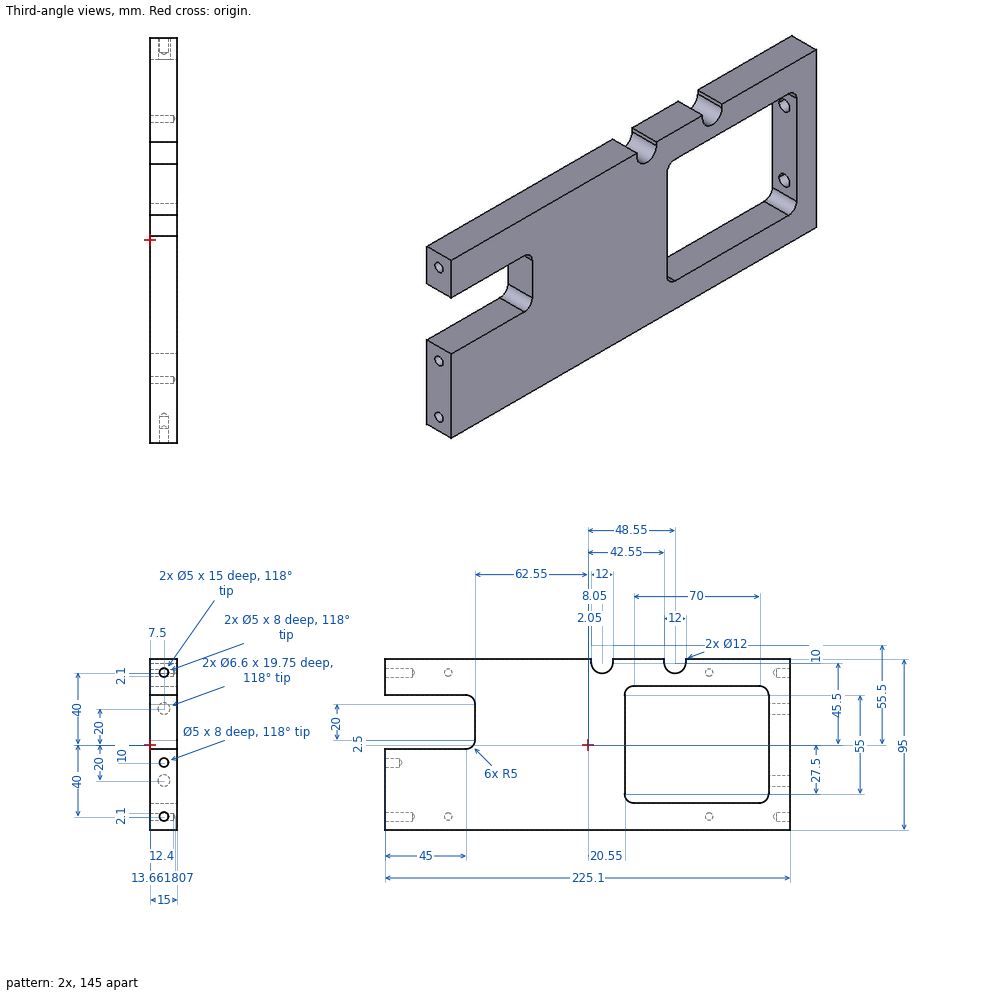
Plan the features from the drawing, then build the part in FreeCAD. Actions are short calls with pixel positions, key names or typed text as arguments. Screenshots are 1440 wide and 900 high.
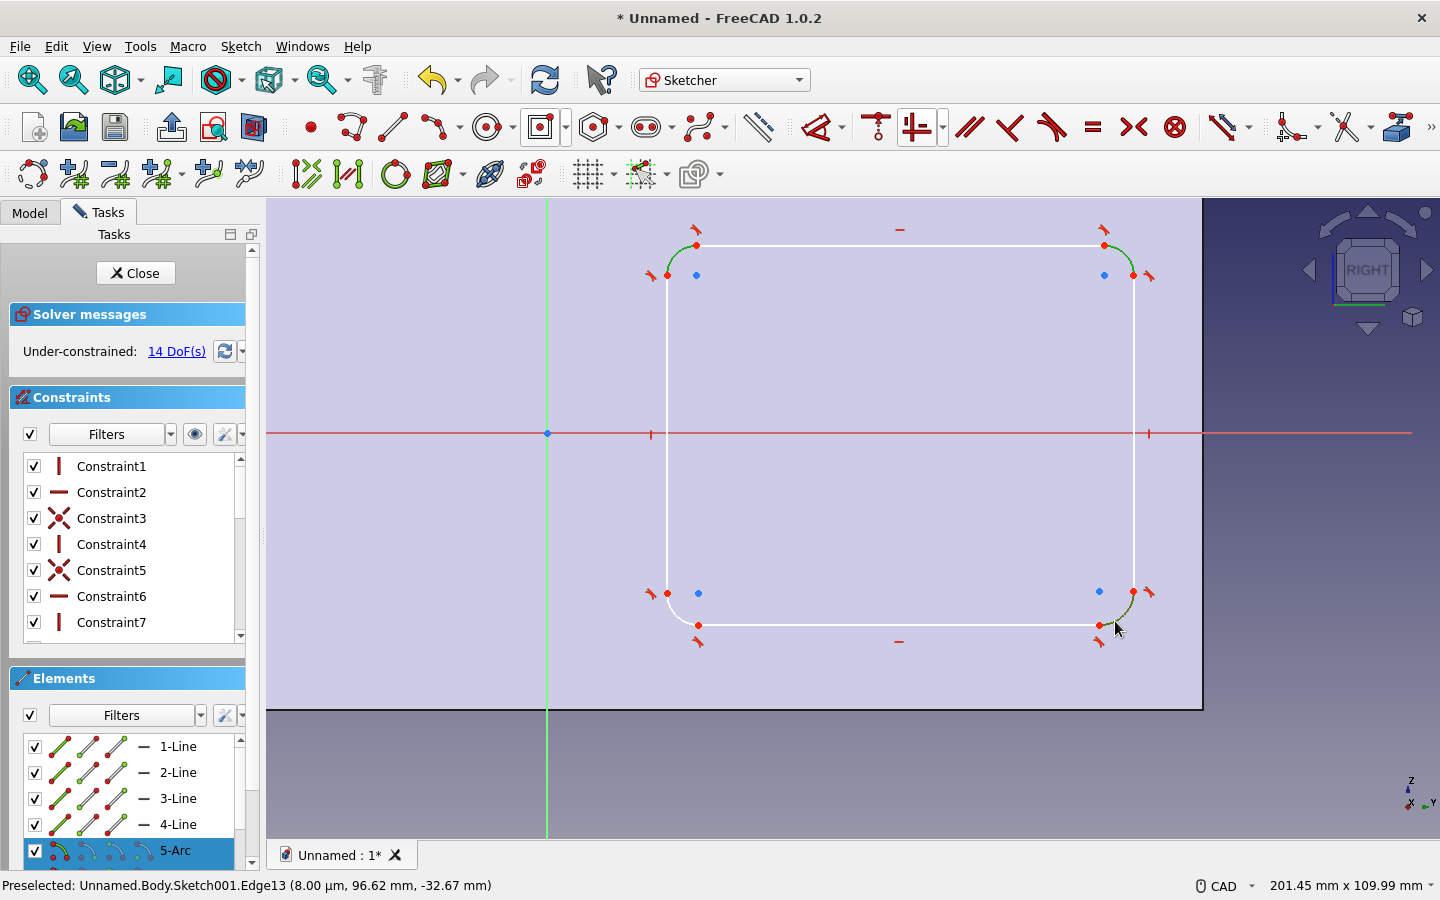
click(671, 608)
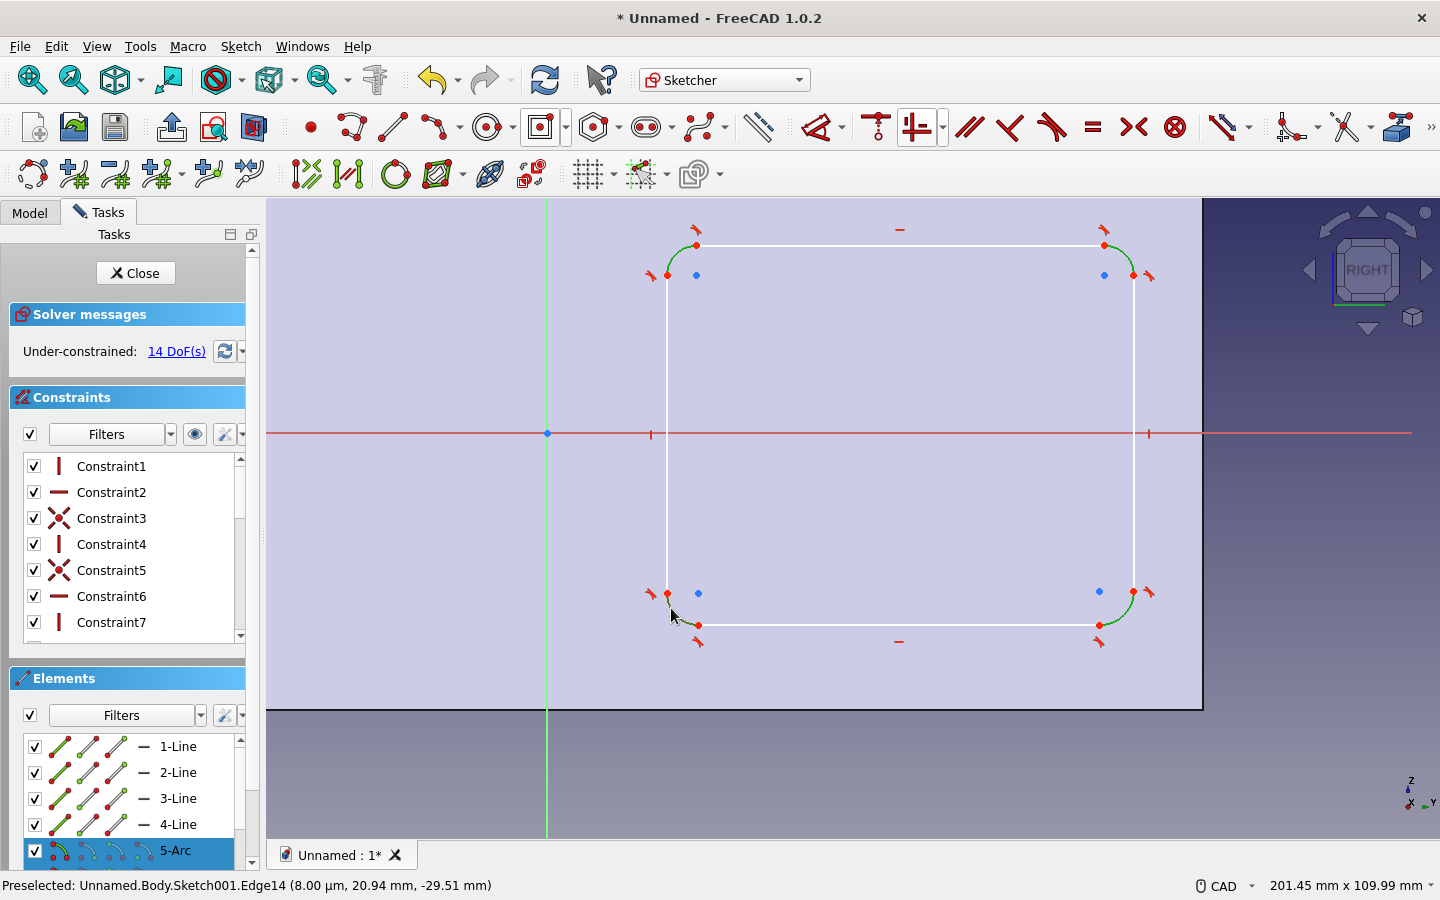
click(1093, 128)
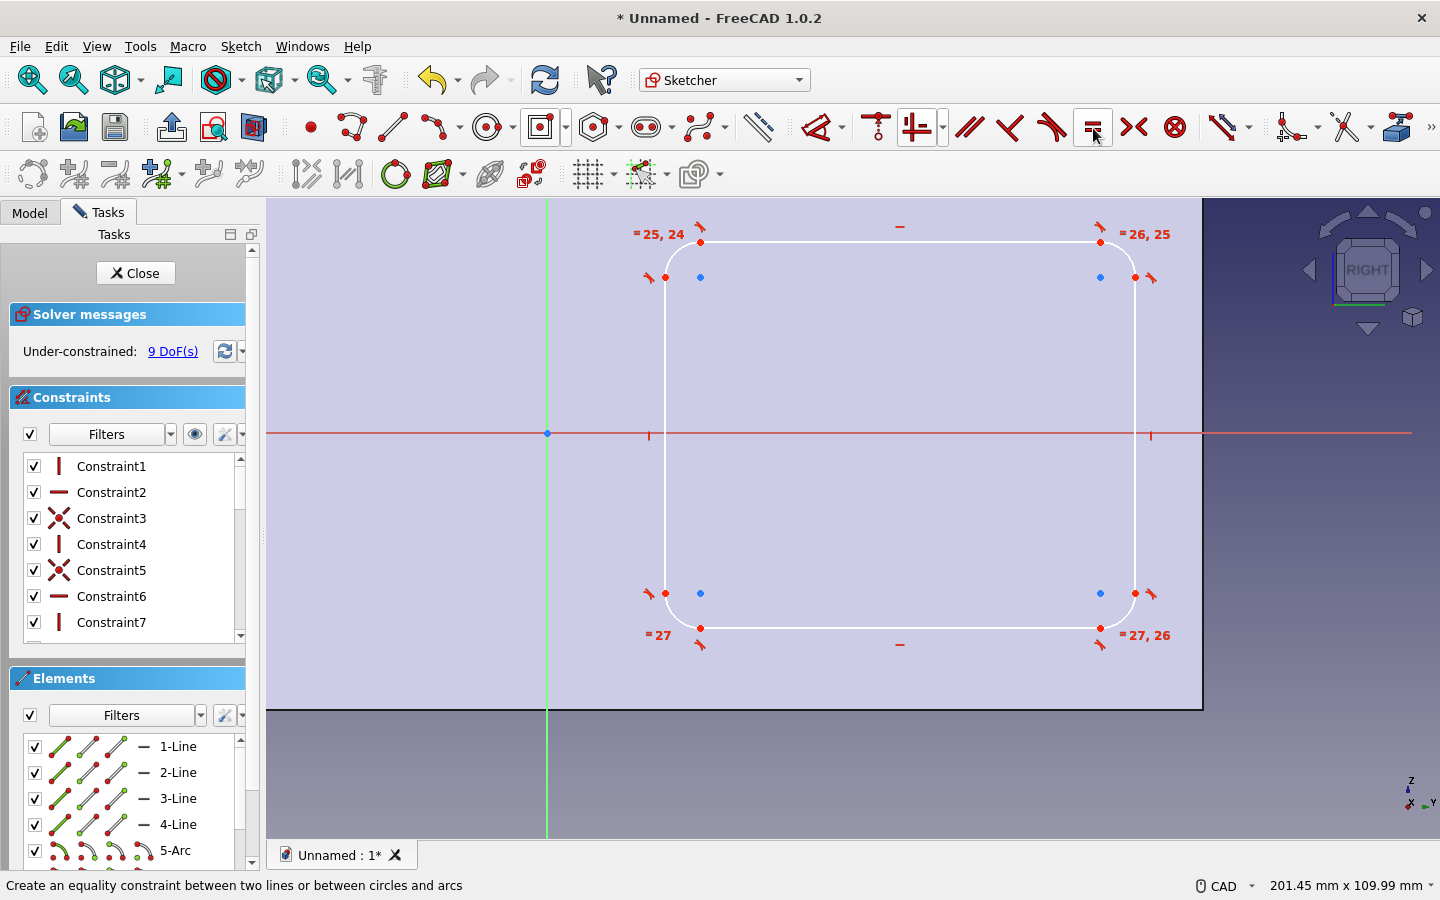
click(816, 128)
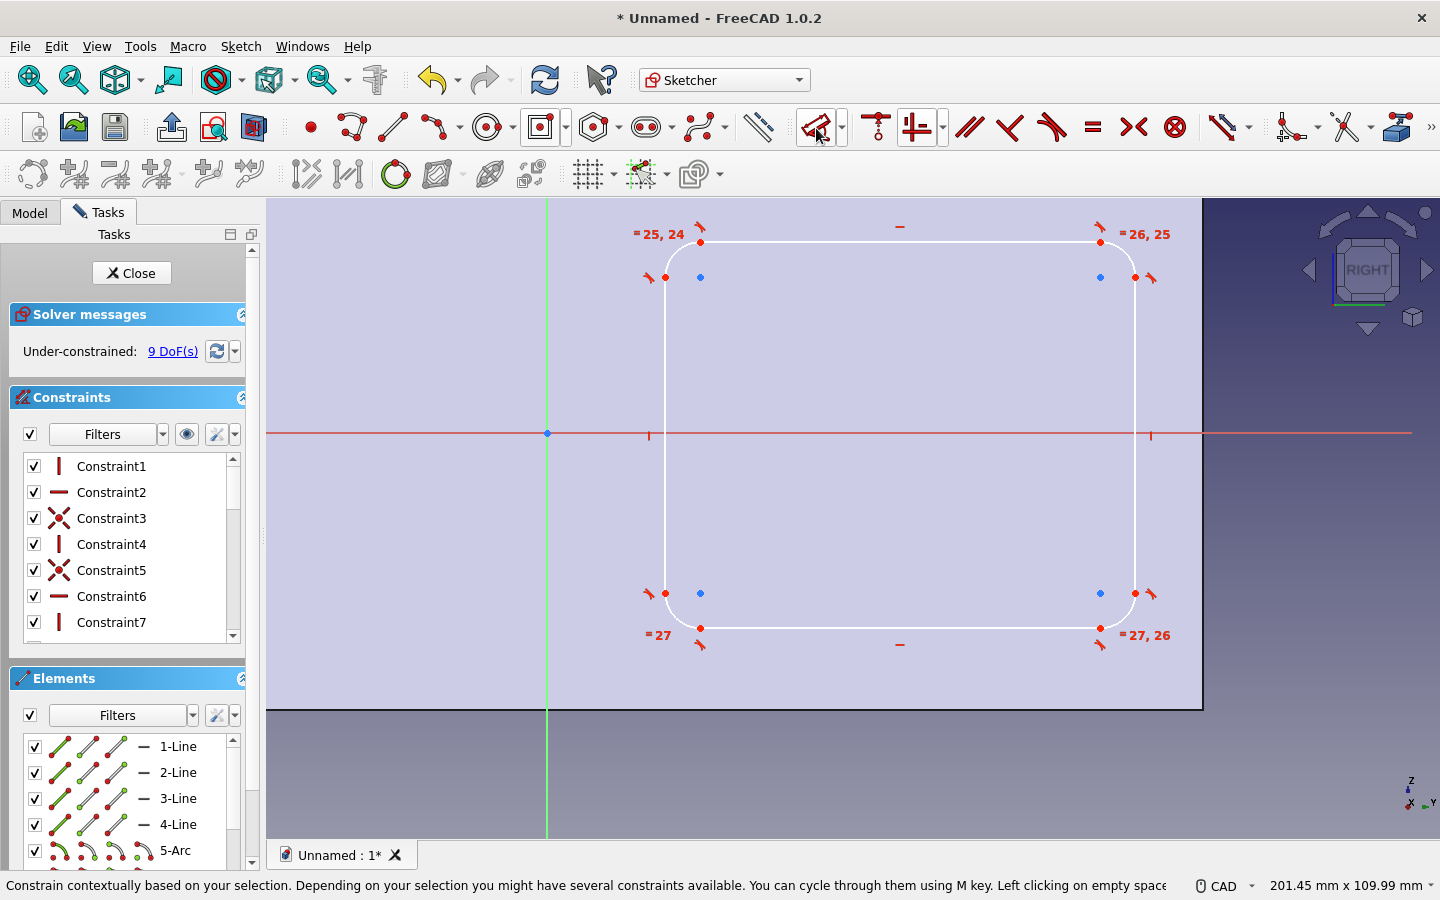
scroll(1116, 622, down, 3)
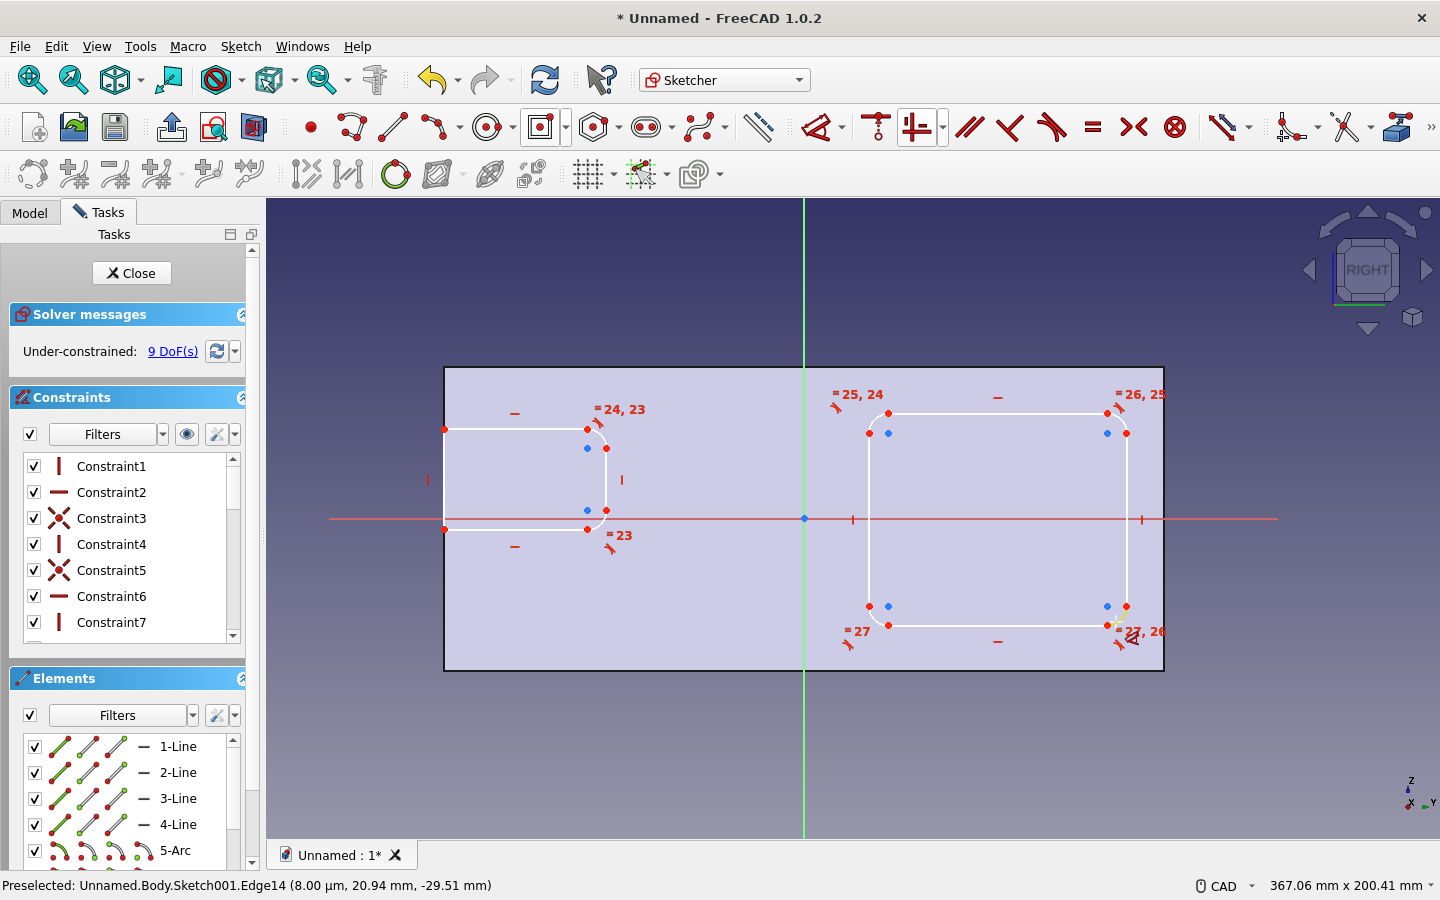
scroll(596, 528, up, 5)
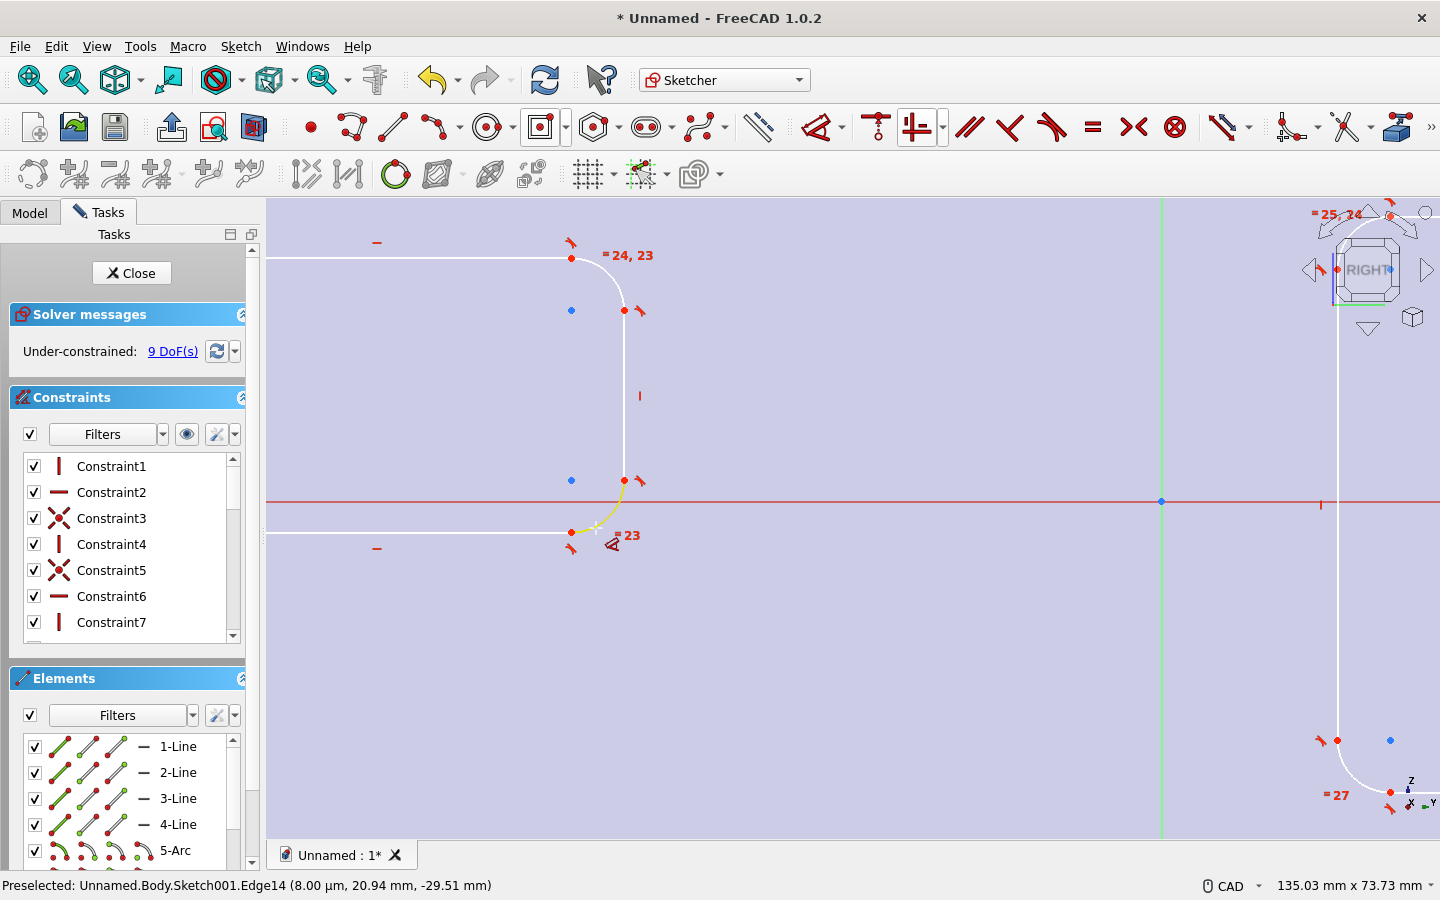
click(596, 527)
click(611, 555)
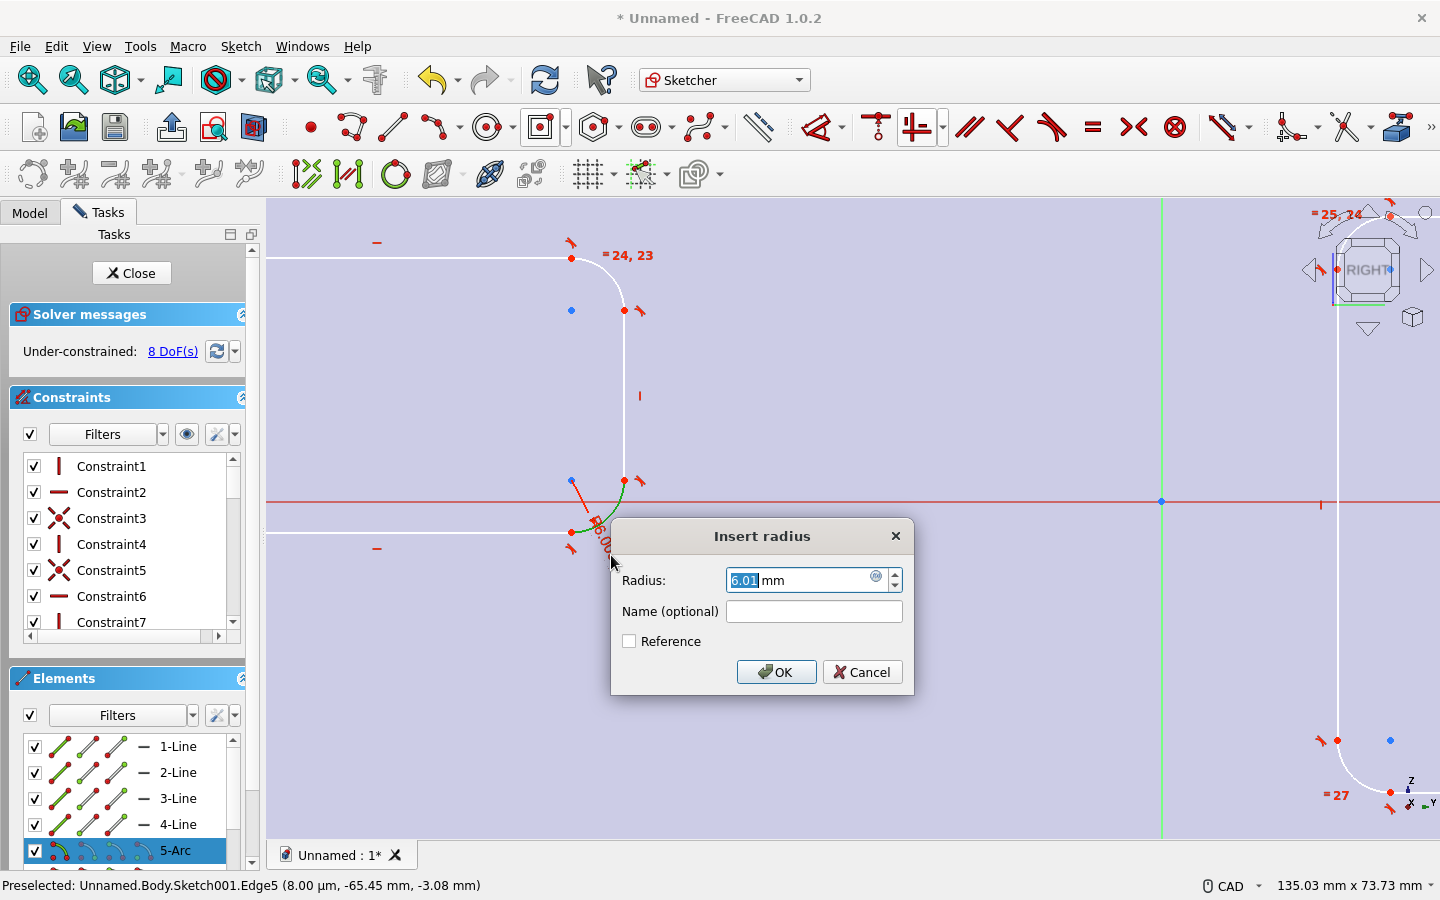
text(5)
key(Return)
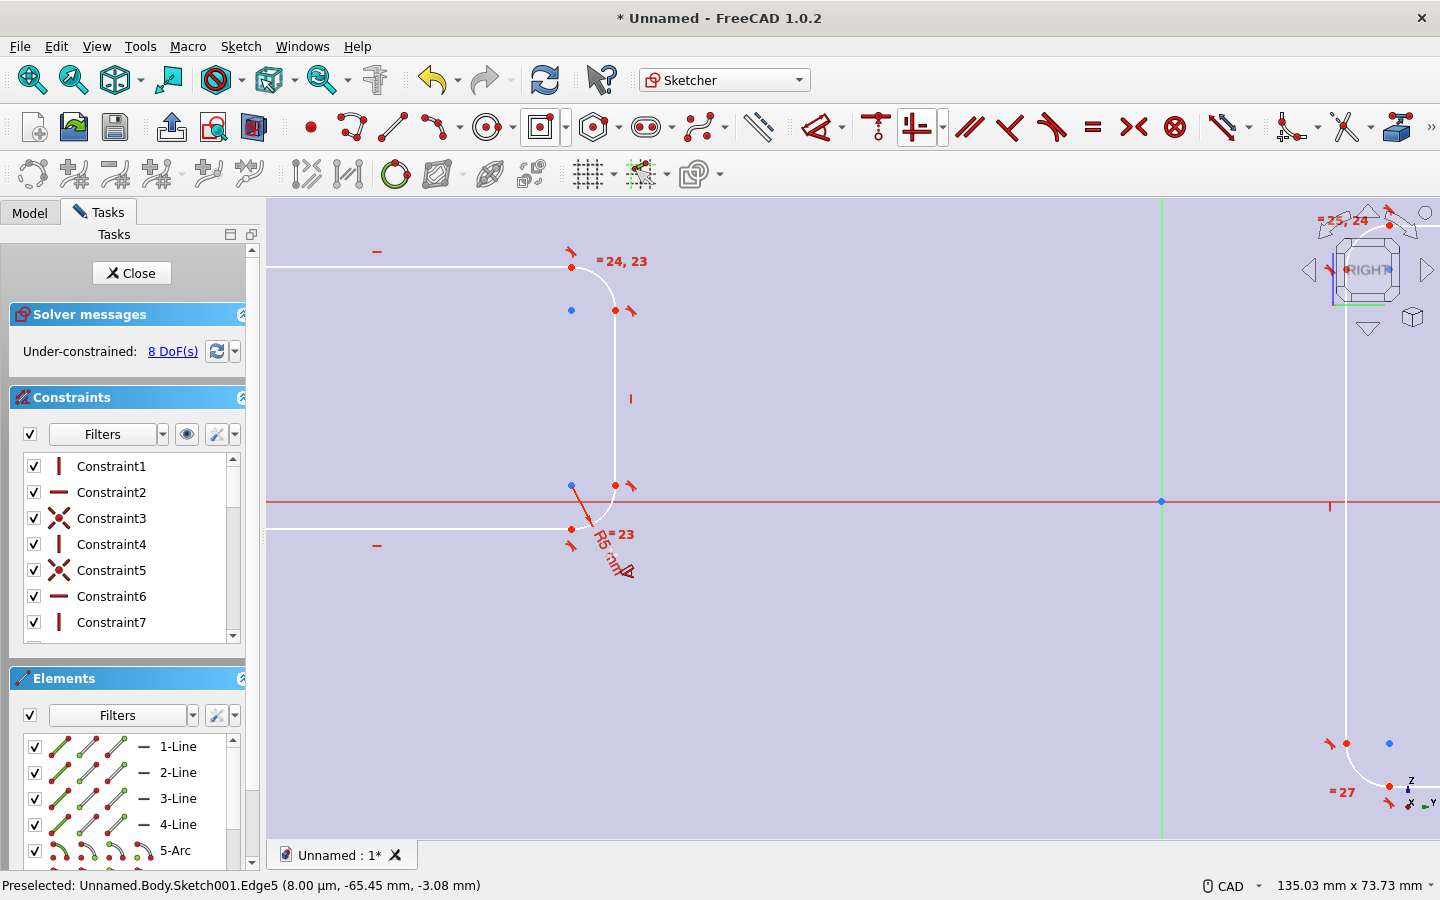
click(615, 363)
click(581, 398)